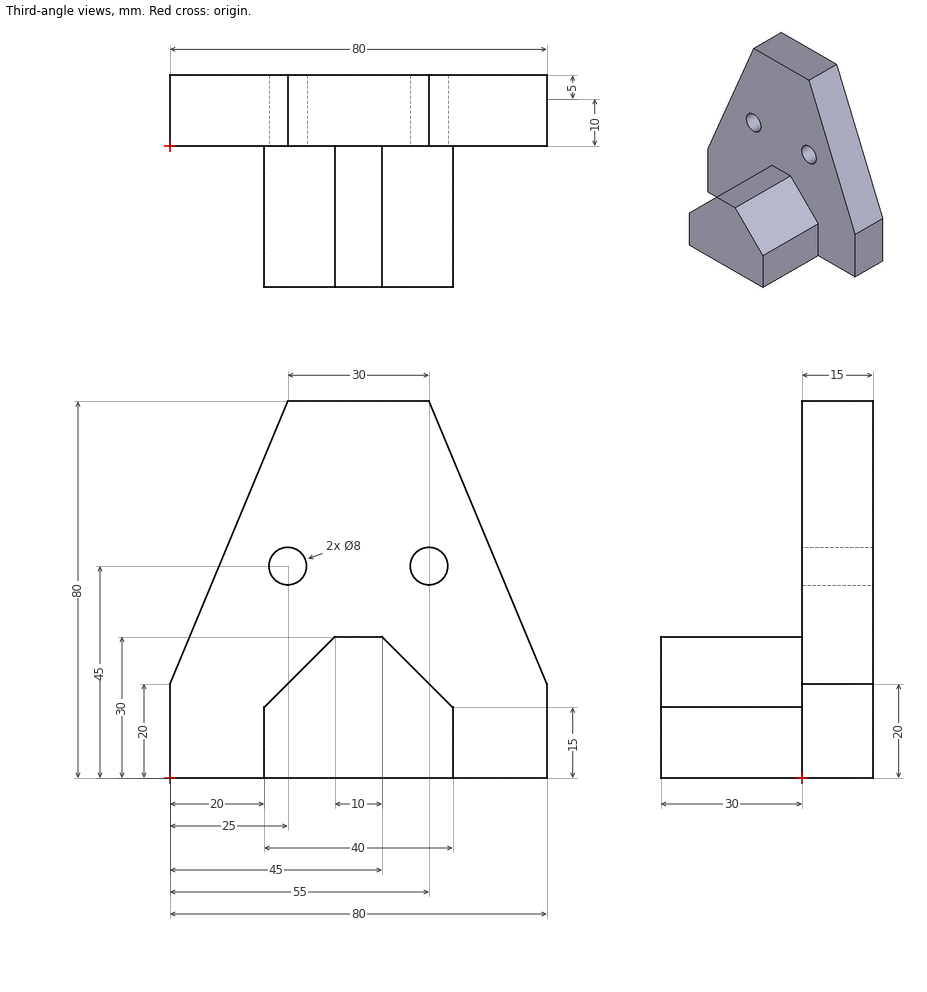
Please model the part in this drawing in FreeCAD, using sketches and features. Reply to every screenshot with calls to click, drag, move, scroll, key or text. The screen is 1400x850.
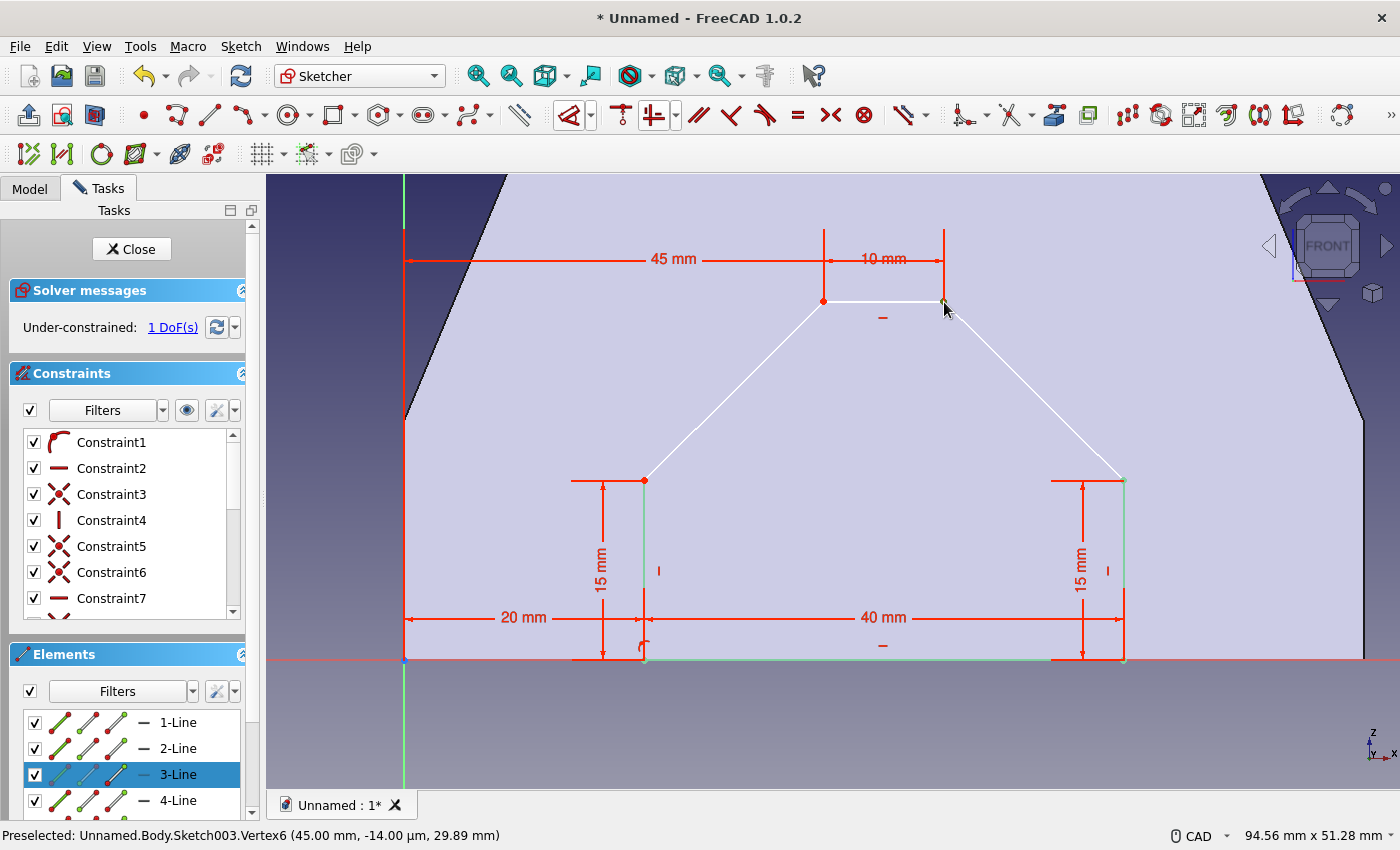
key(i)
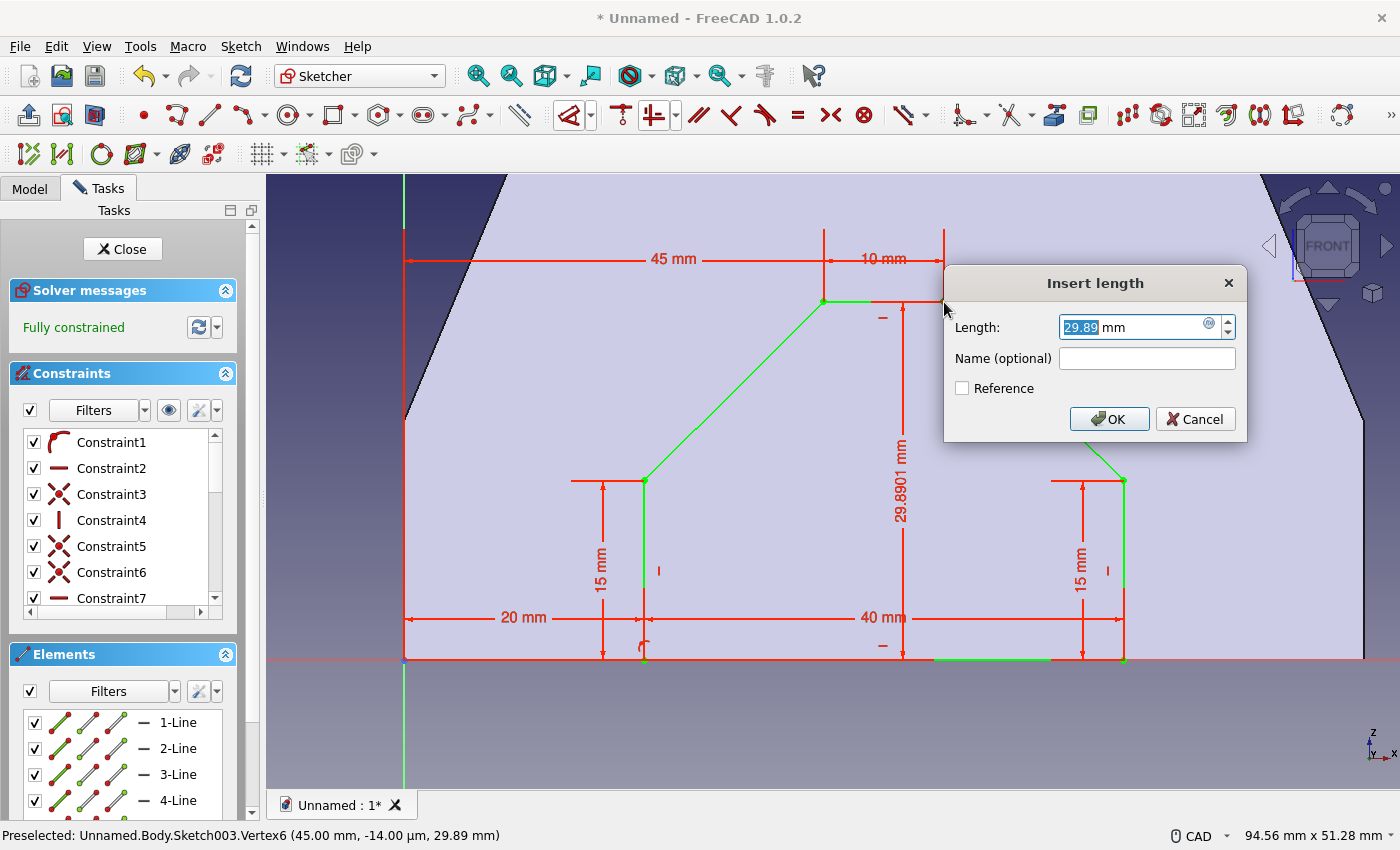
text(30)
key(Return)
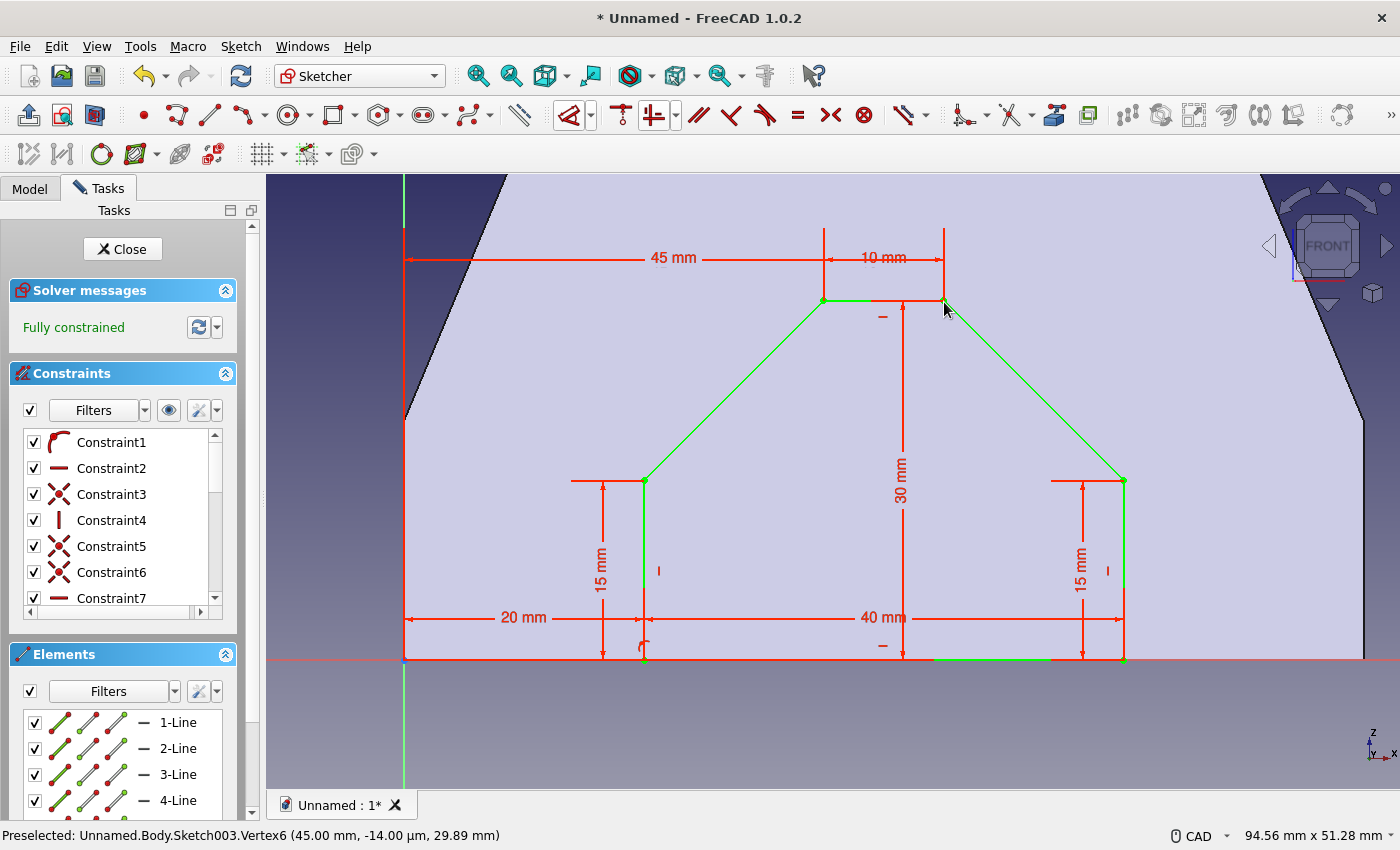
click(123, 249)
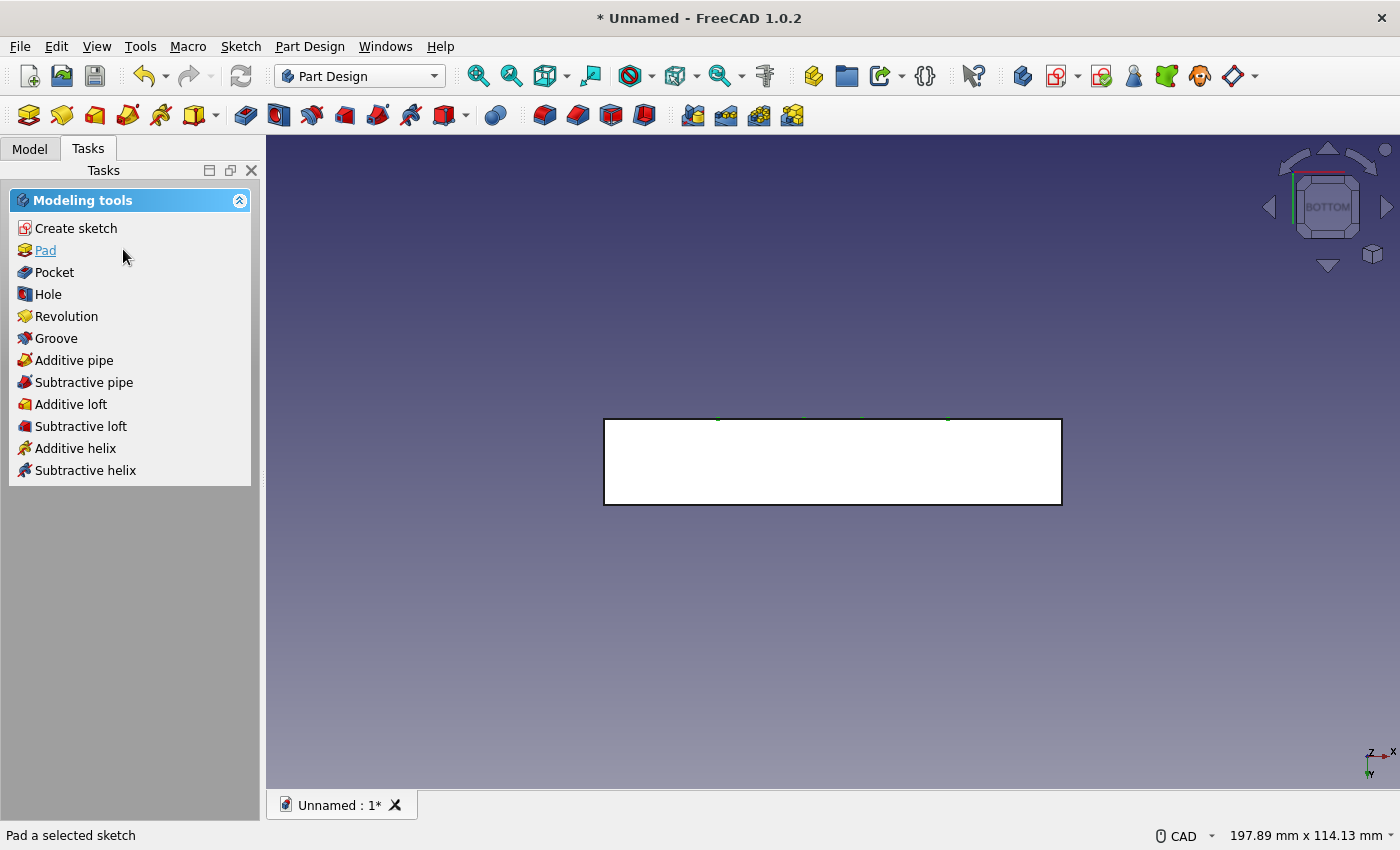
click(29, 116)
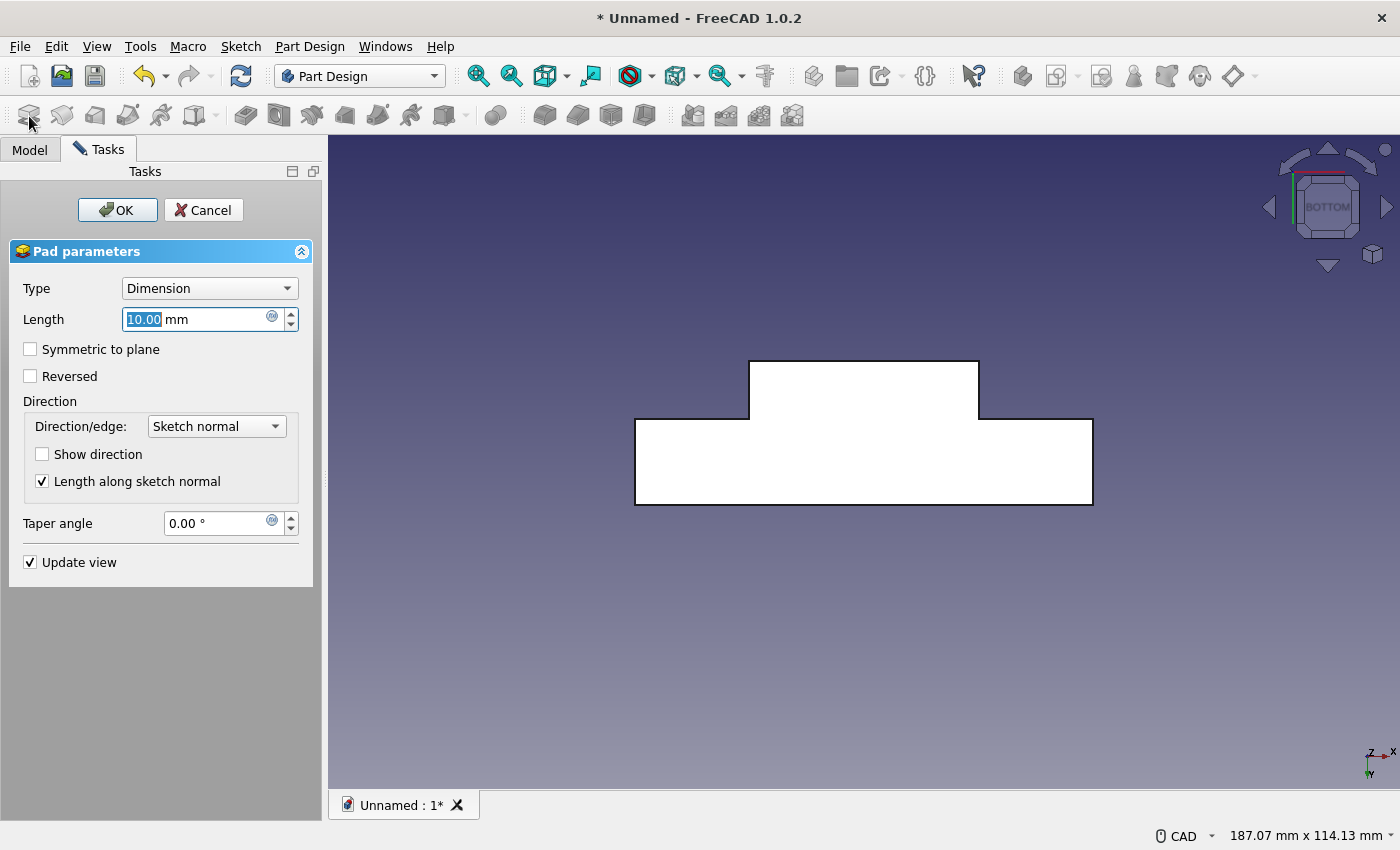
text(30)
key(Tab)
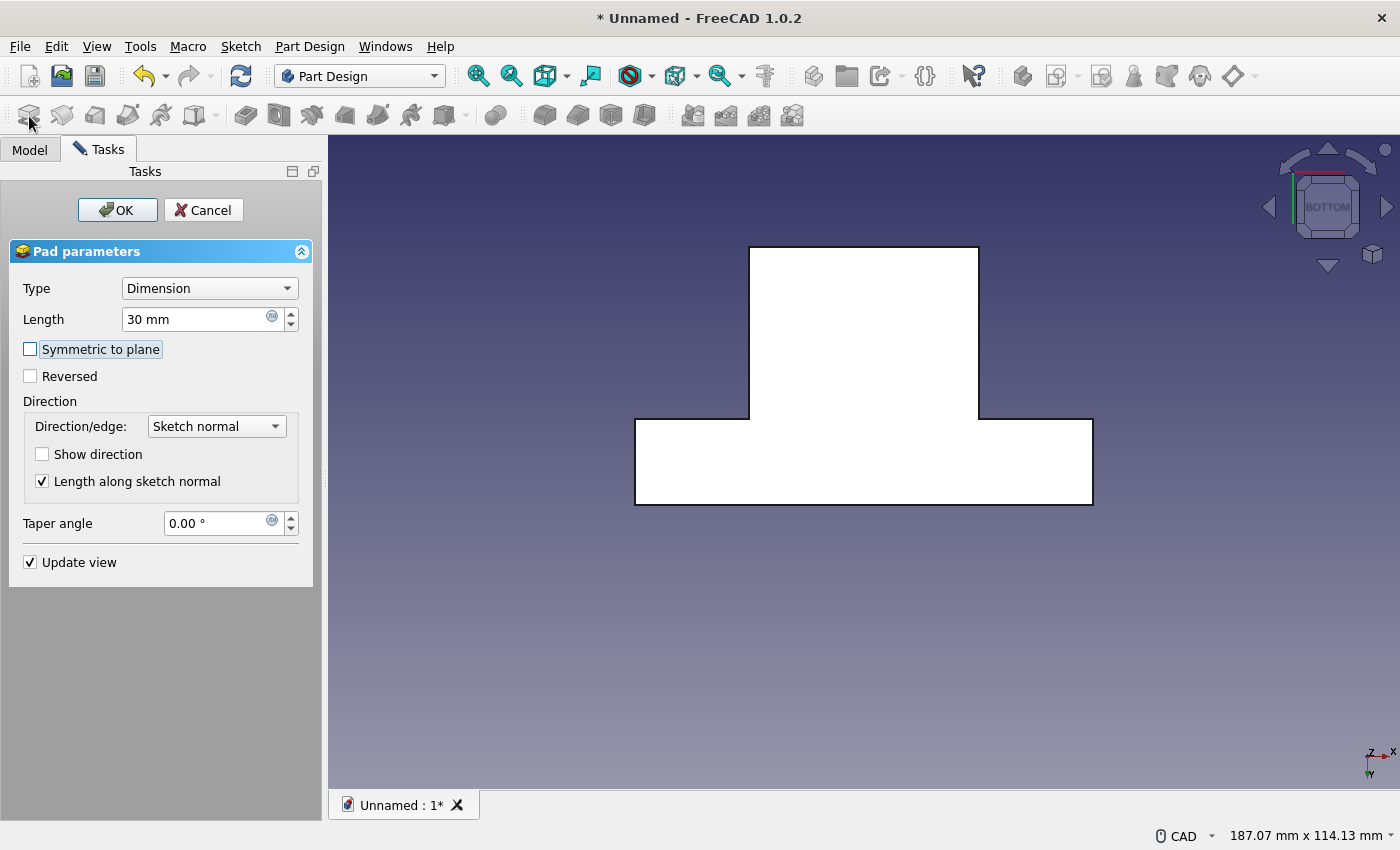
click(118, 210)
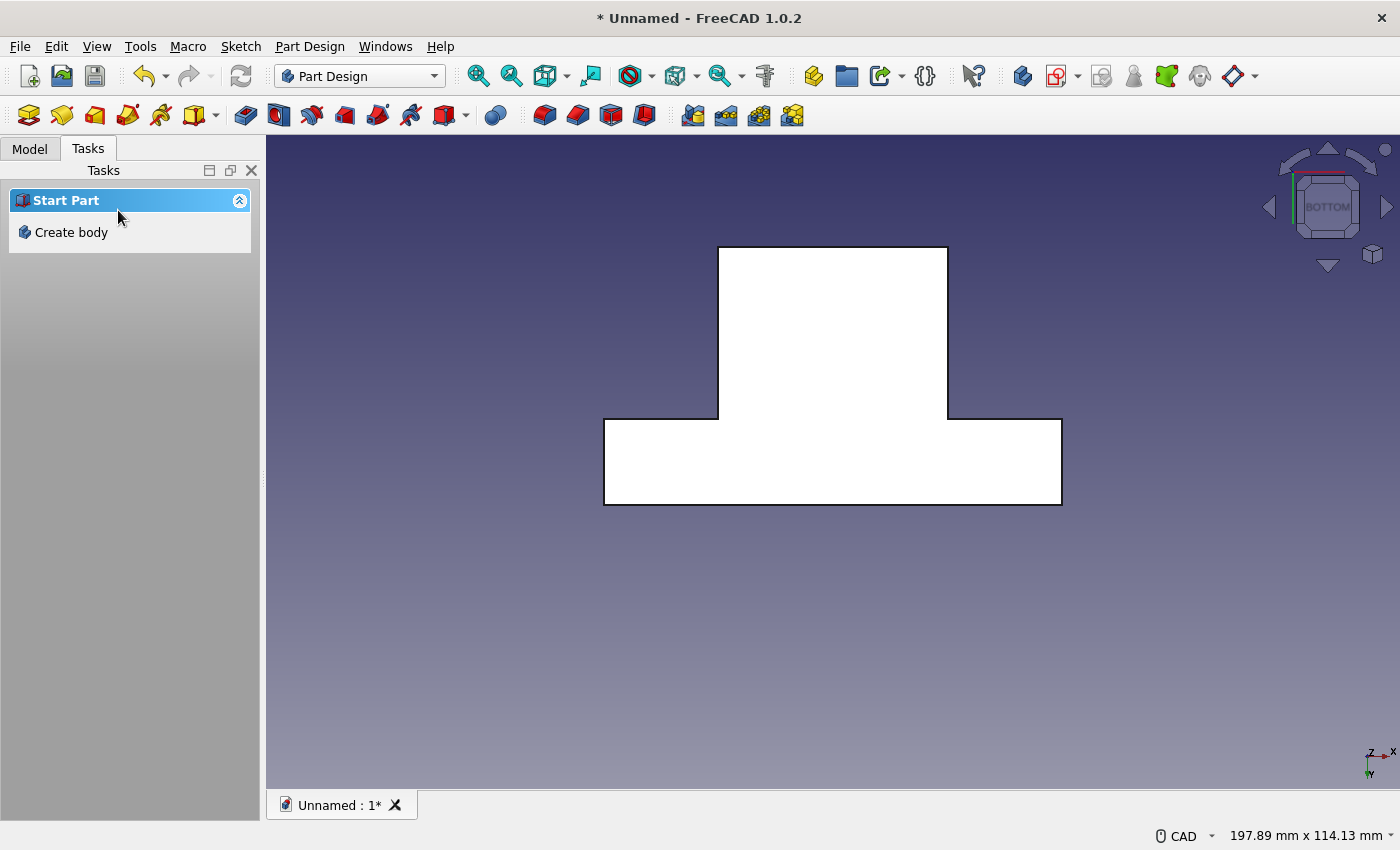
click(479, 76)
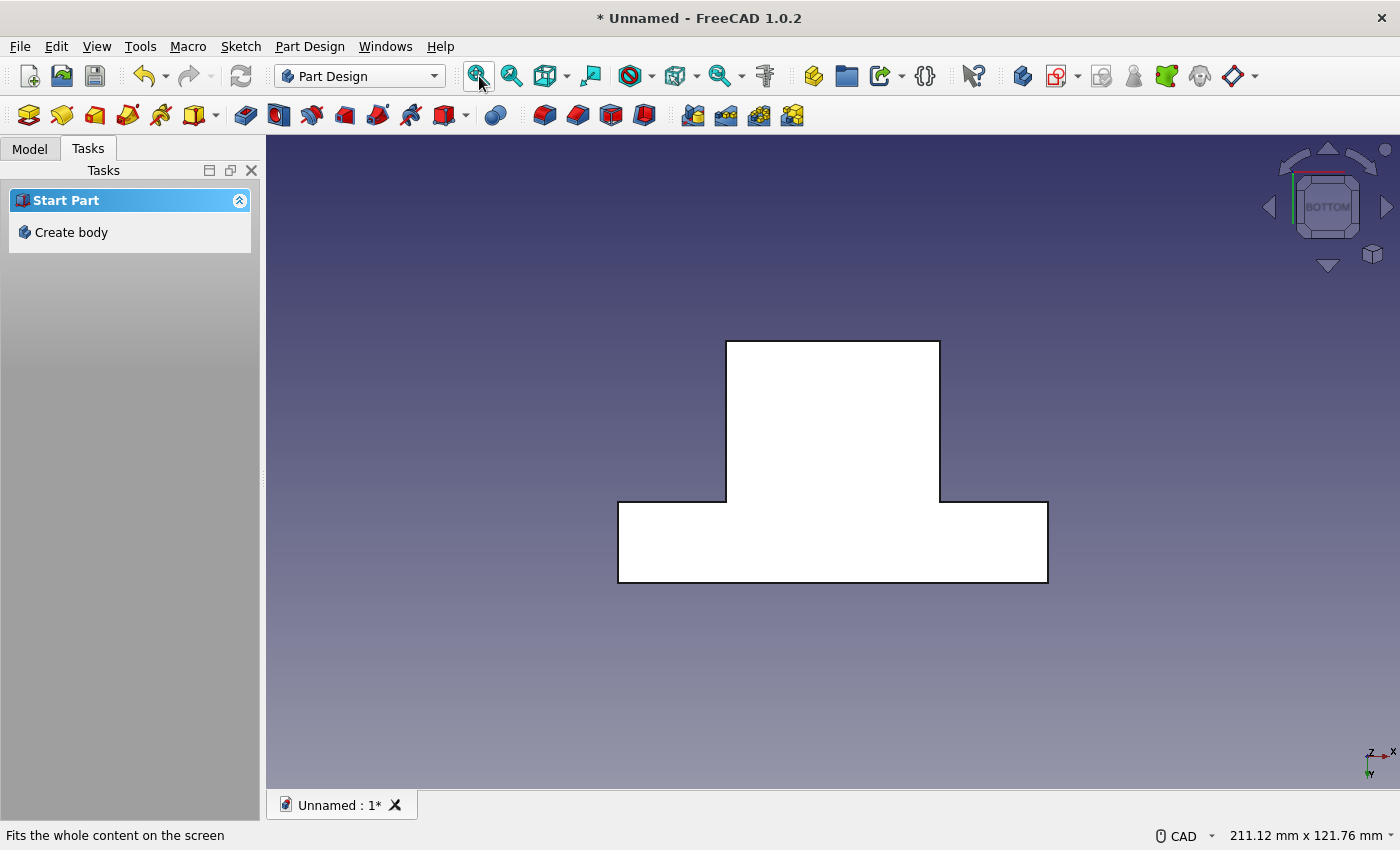
click(1056, 76)